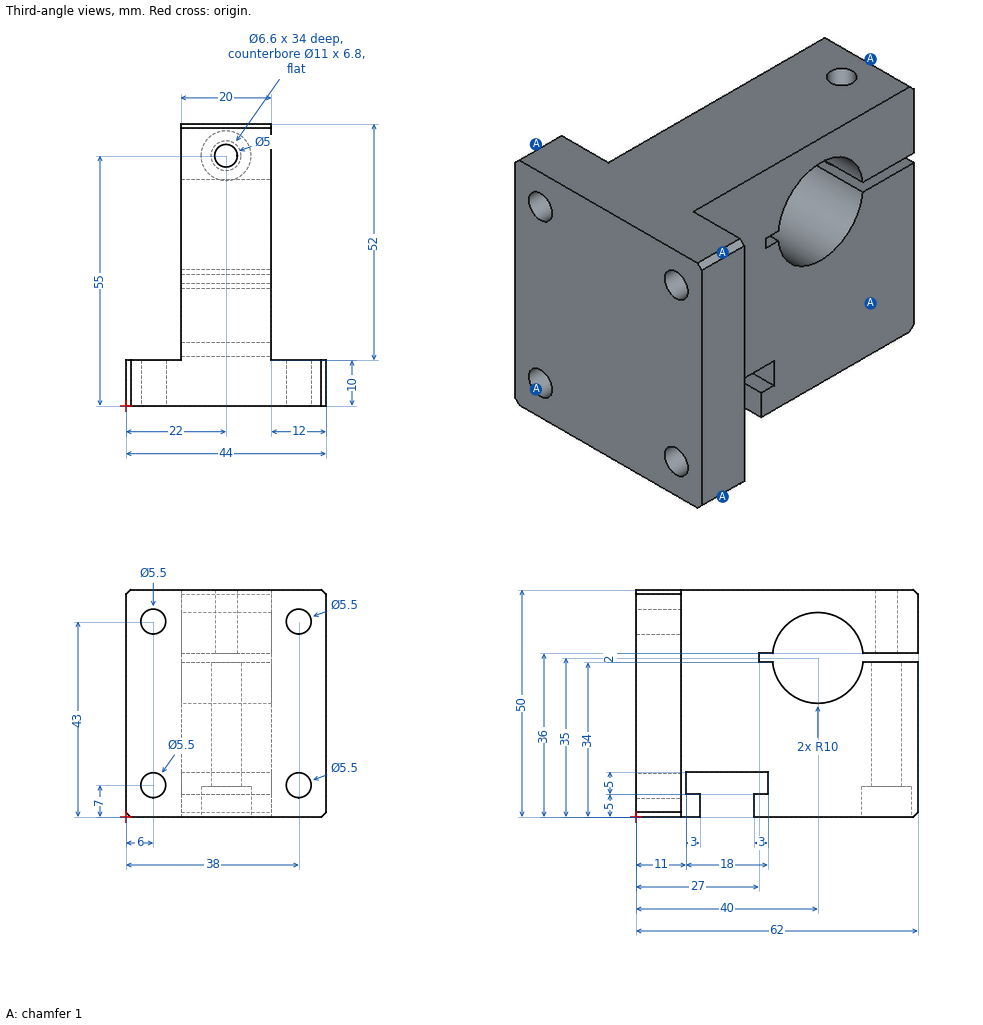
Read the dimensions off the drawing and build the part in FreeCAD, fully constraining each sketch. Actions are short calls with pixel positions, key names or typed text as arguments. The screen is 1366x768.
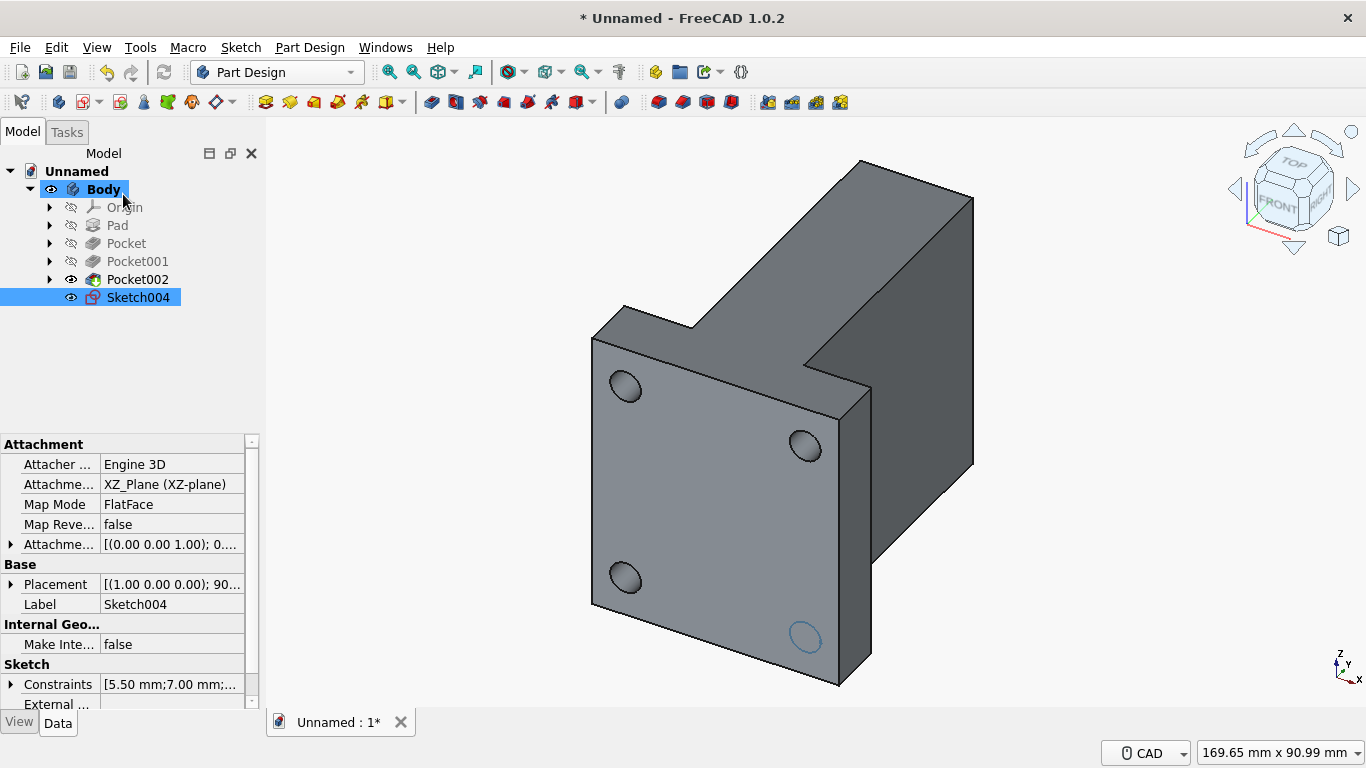
click(432, 102)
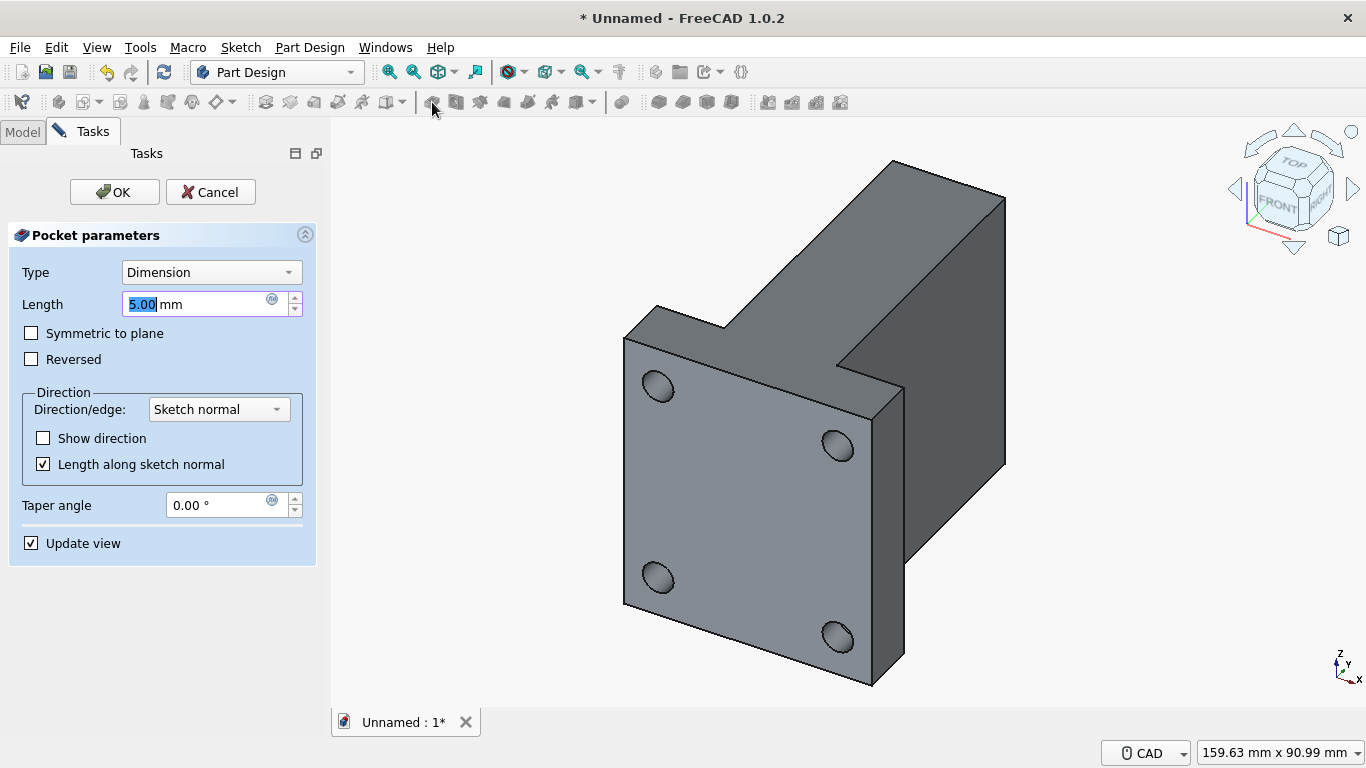
click(212, 272)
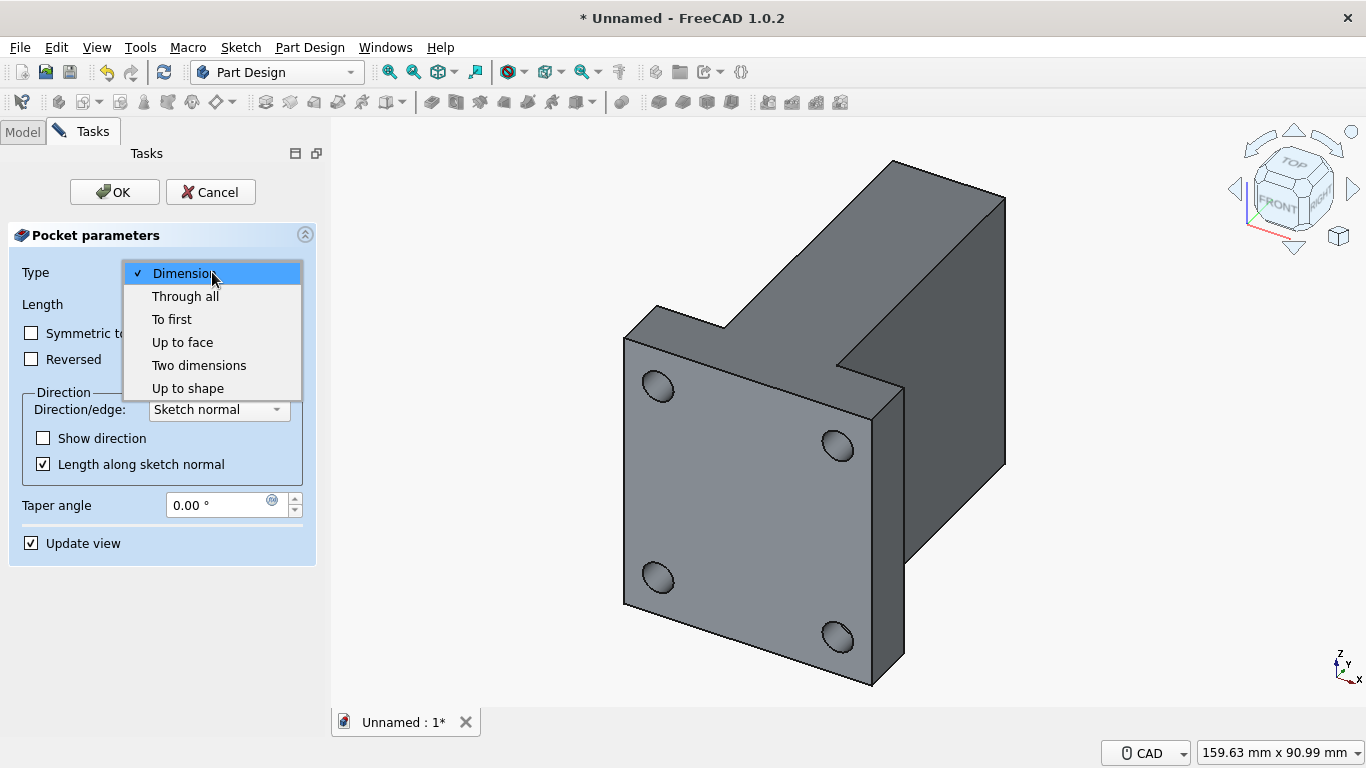
click(212, 320)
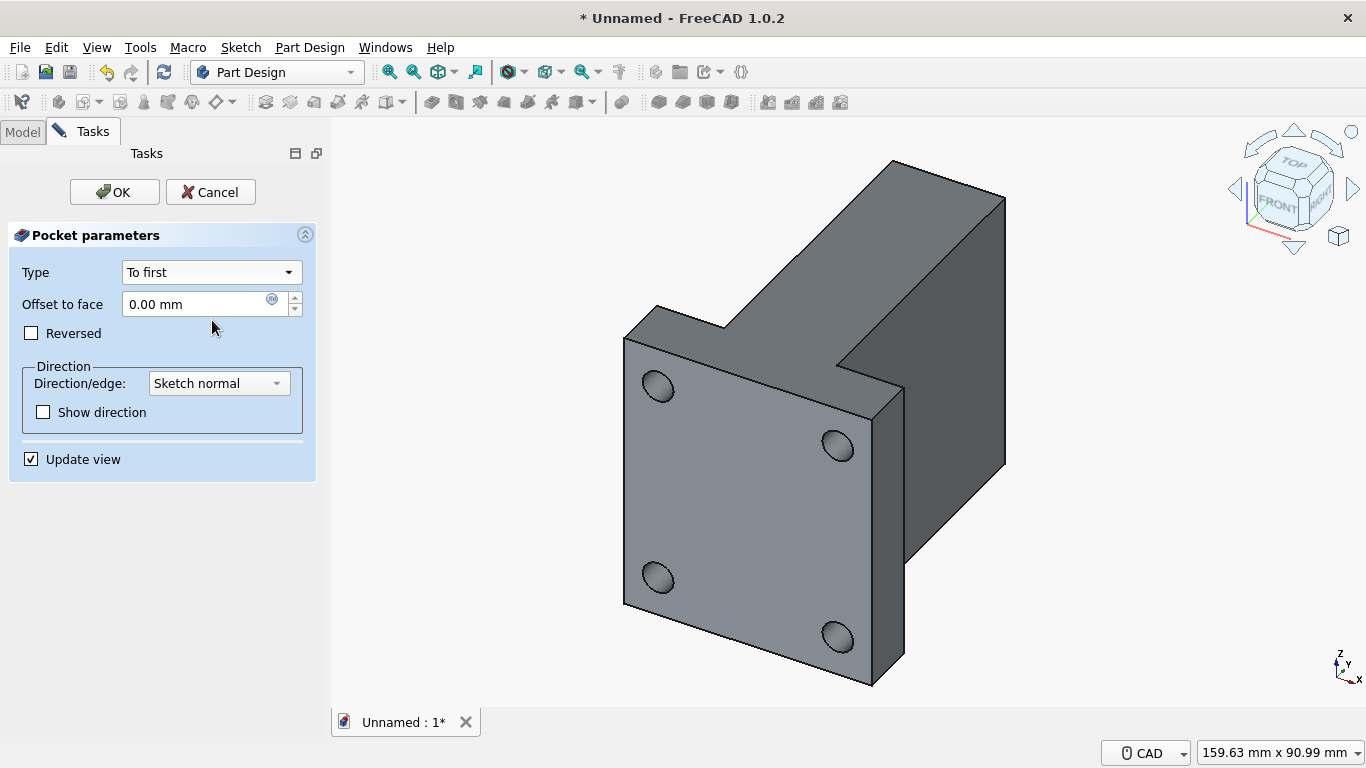
click(115, 192)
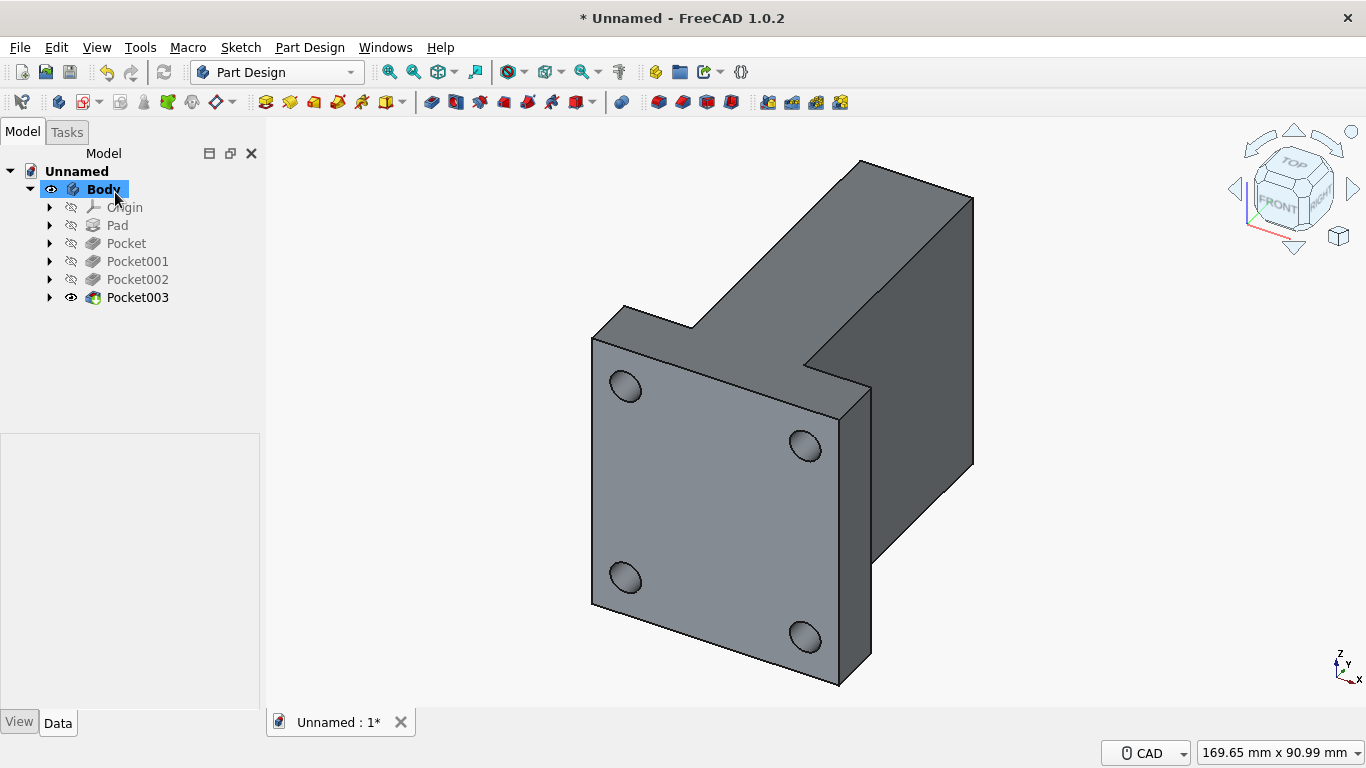
key(6)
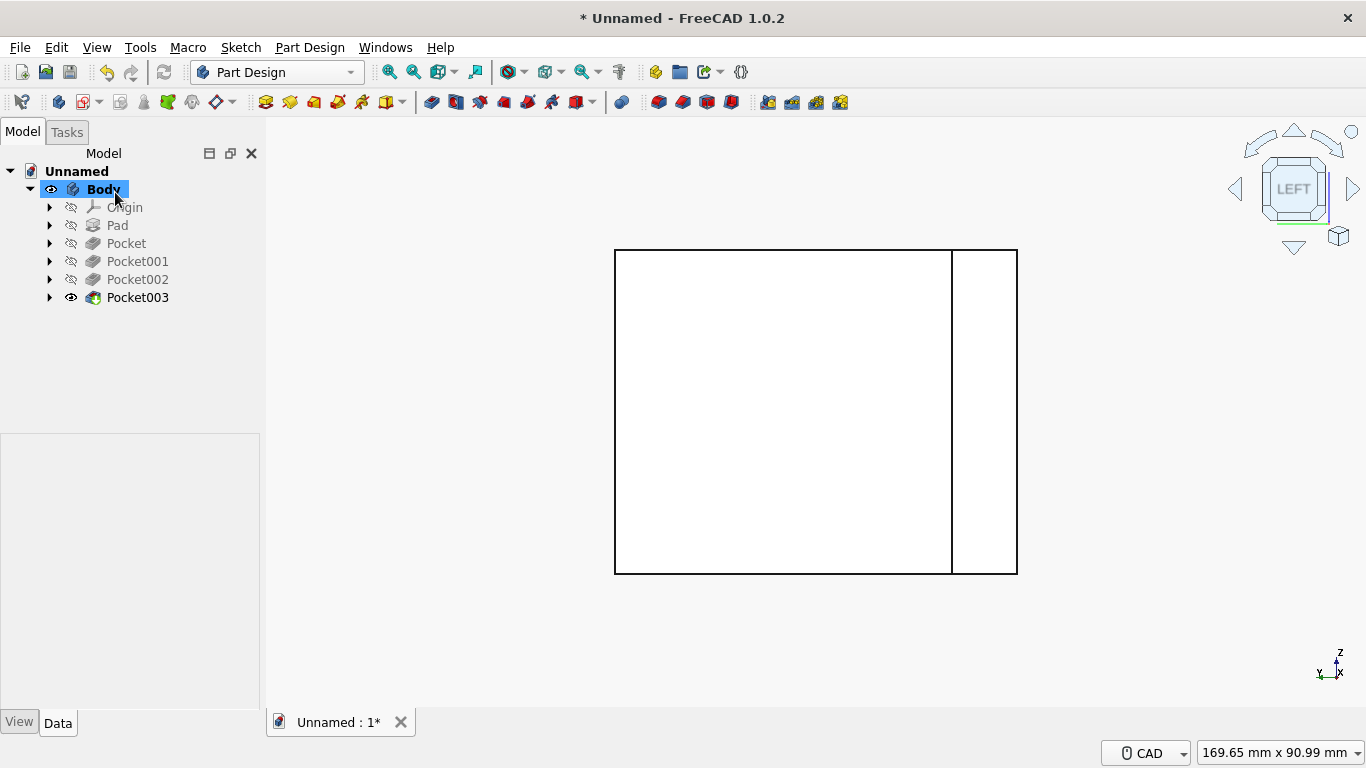
click(784, 411)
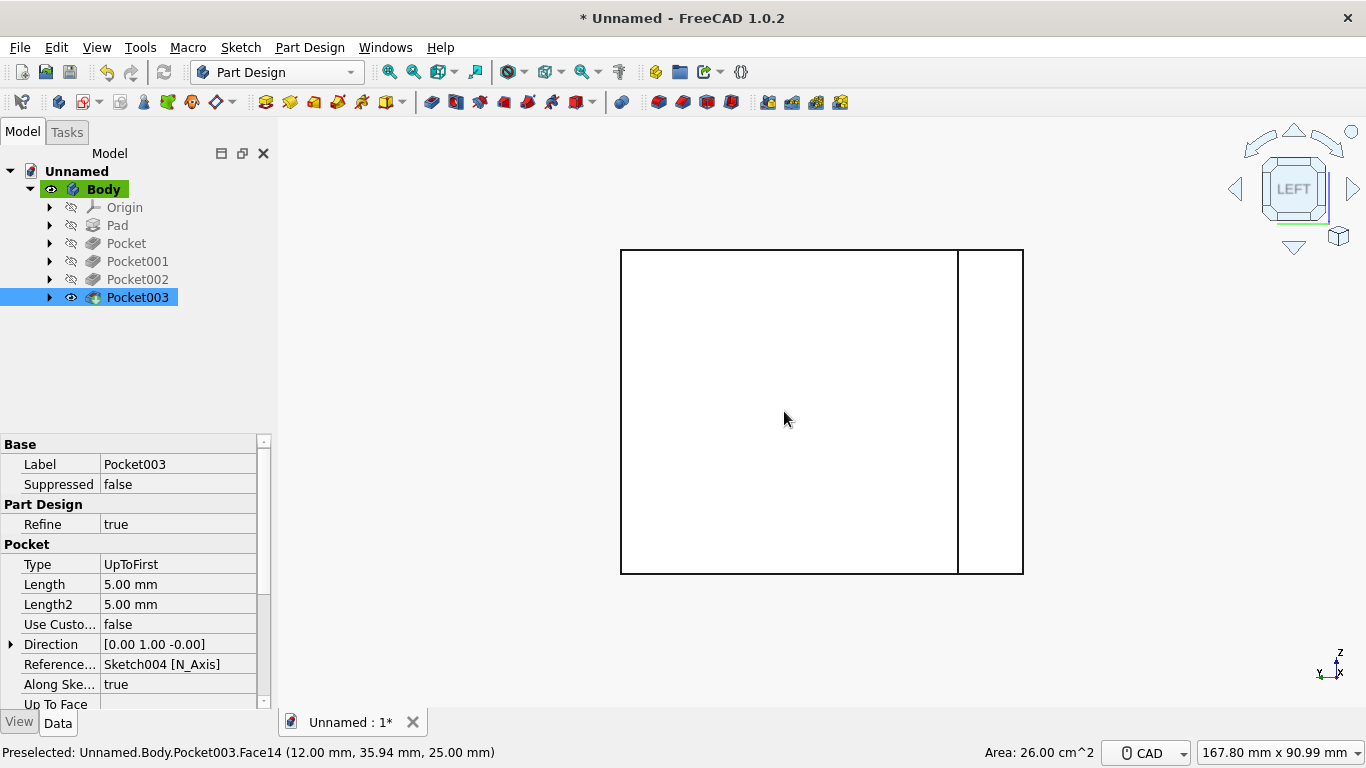
click(84, 102)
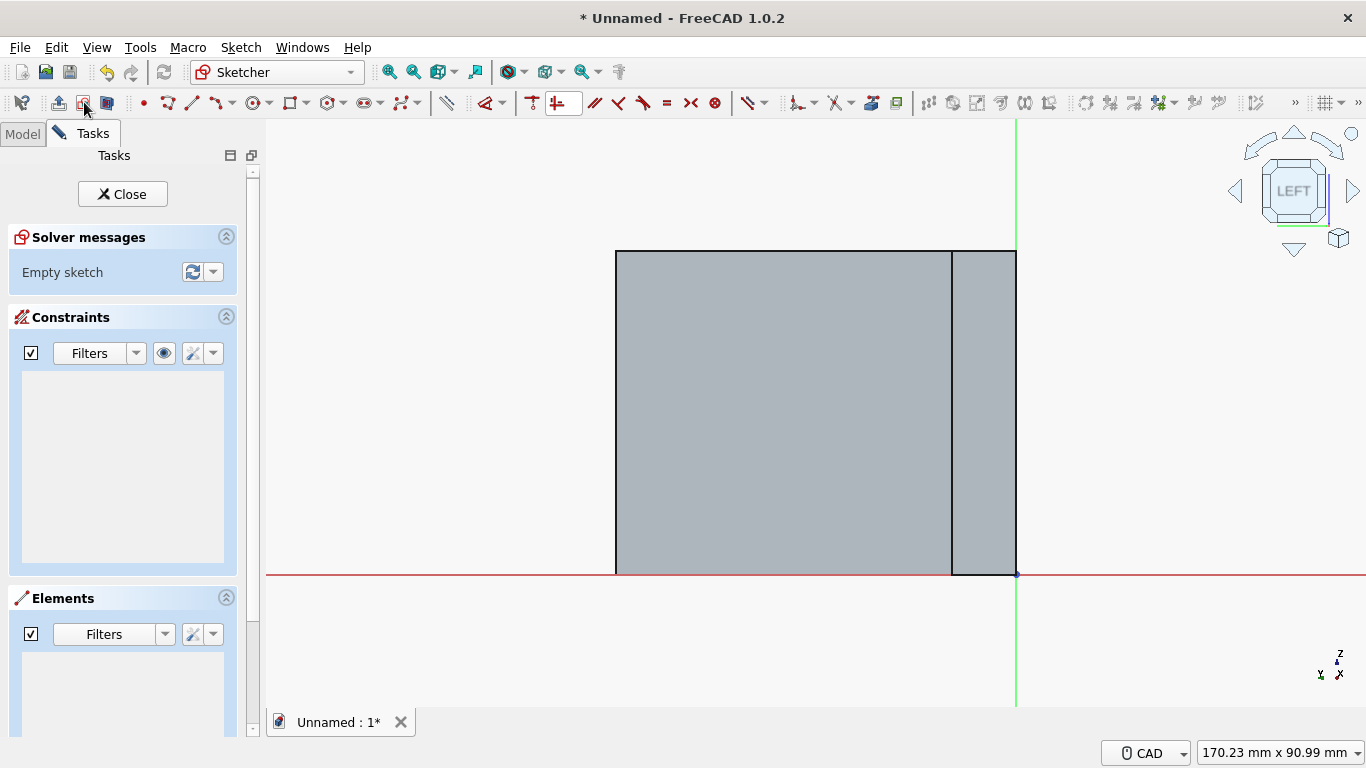
click(168, 104)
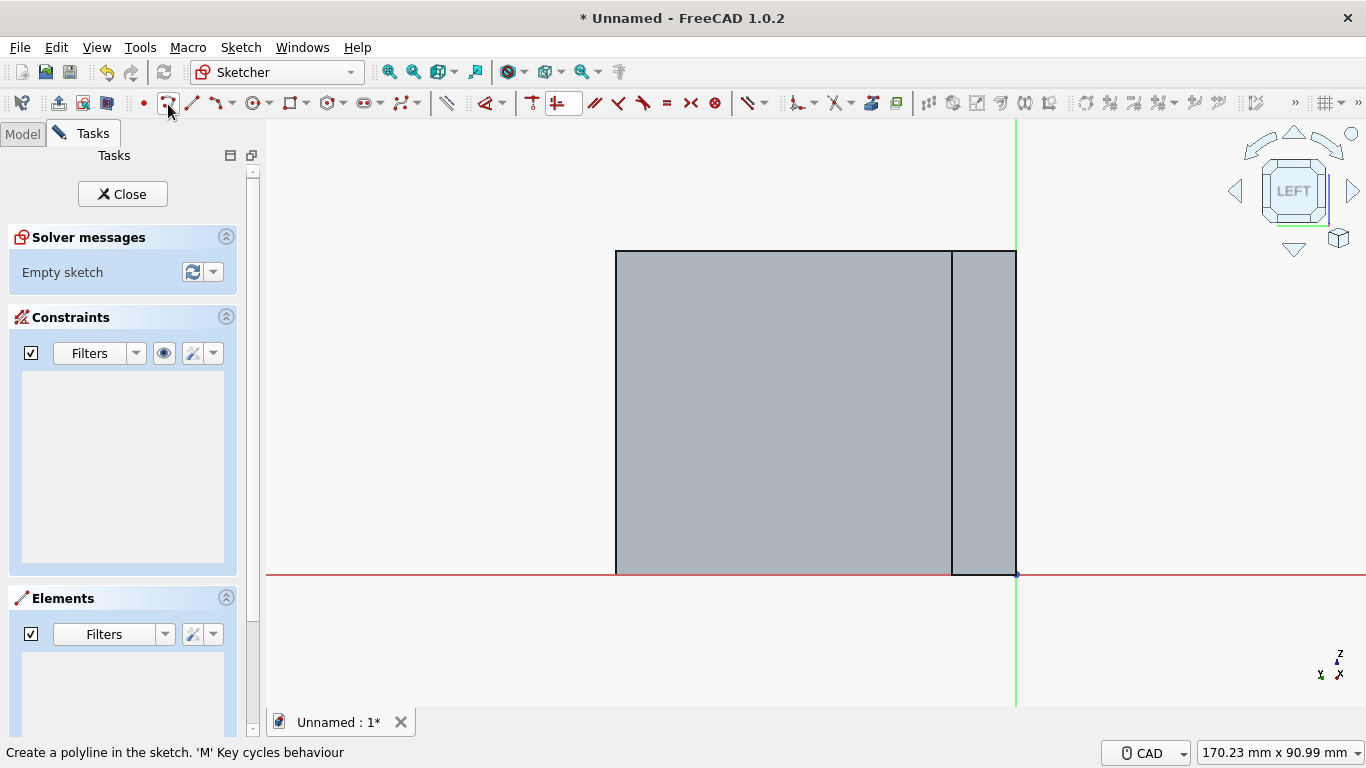
click(822, 355)
click(842, 355)